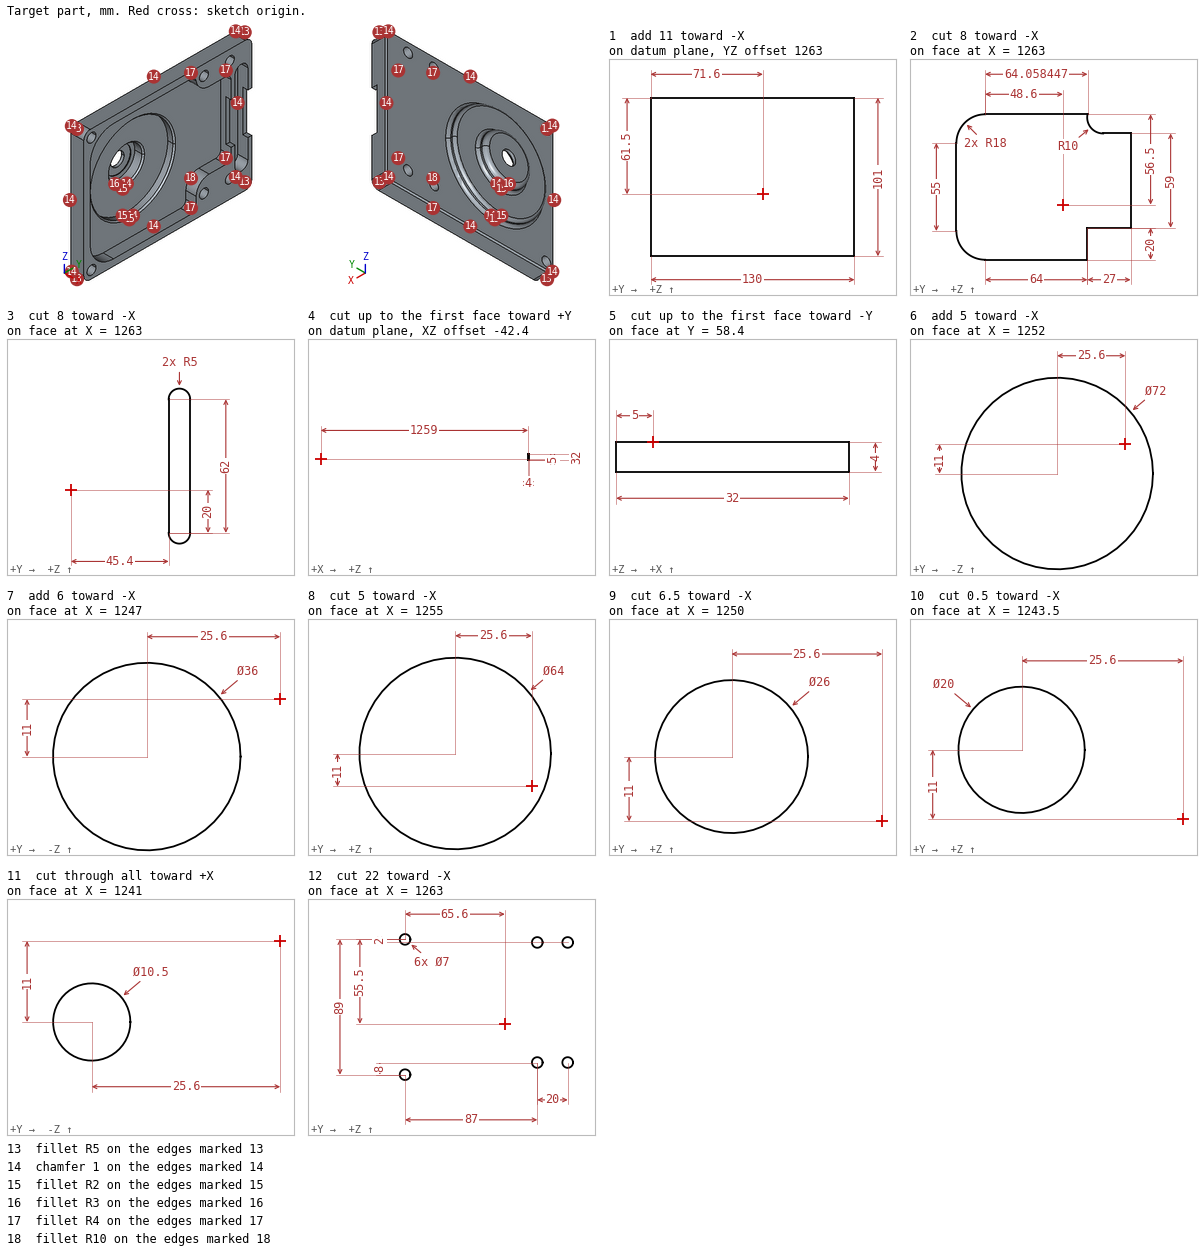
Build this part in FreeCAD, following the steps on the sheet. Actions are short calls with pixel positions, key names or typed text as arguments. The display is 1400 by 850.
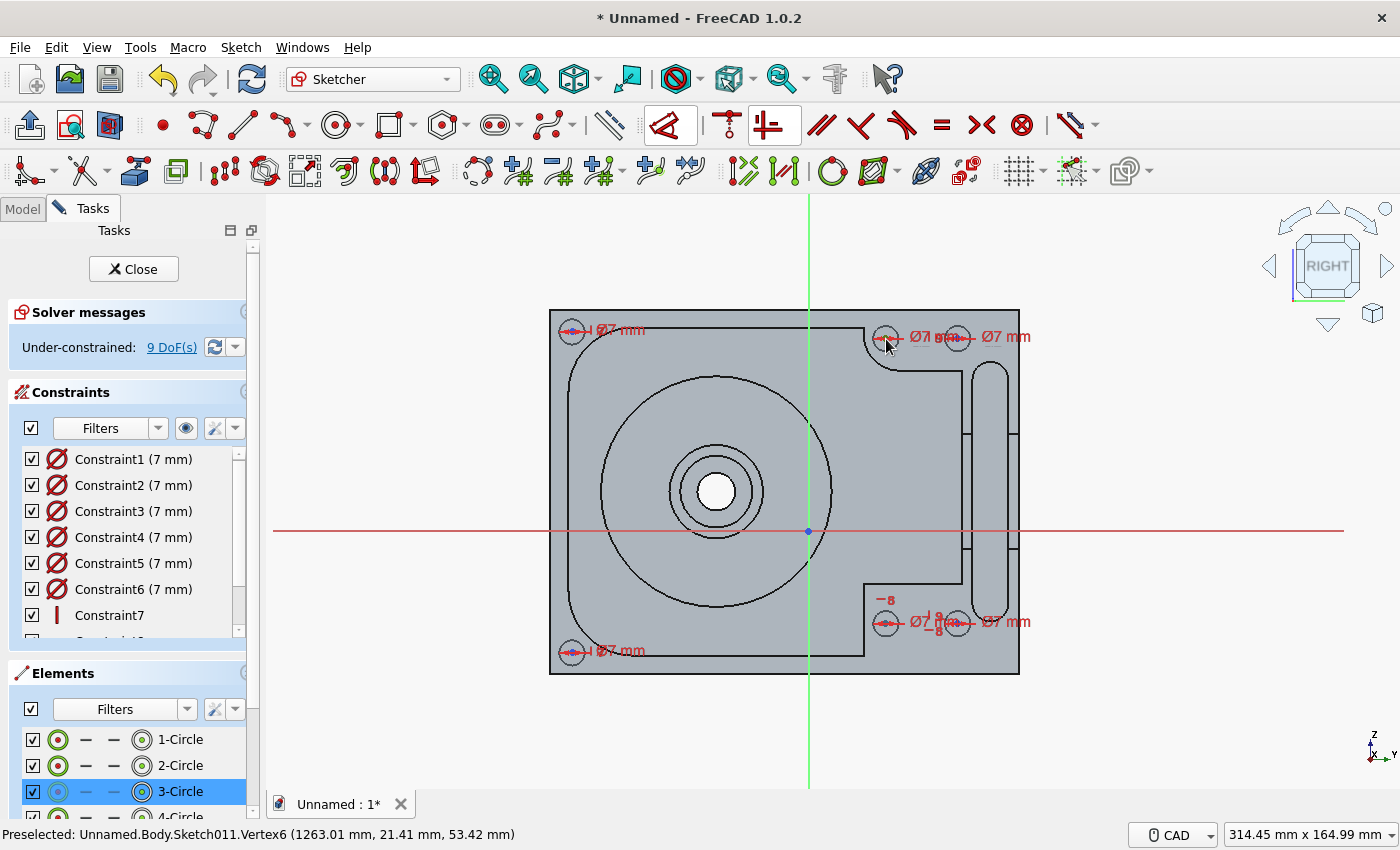
key(v)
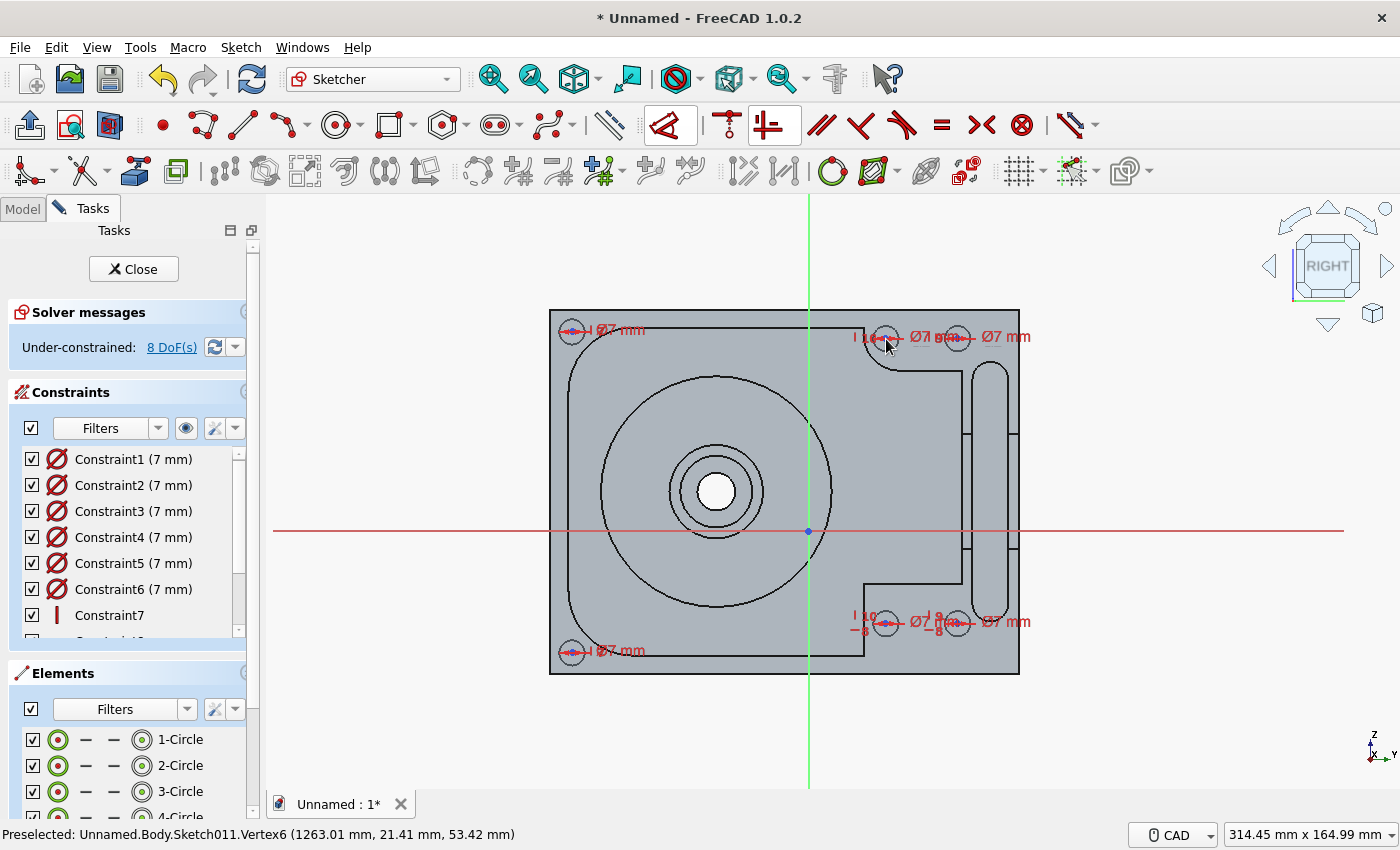
click(958, 339)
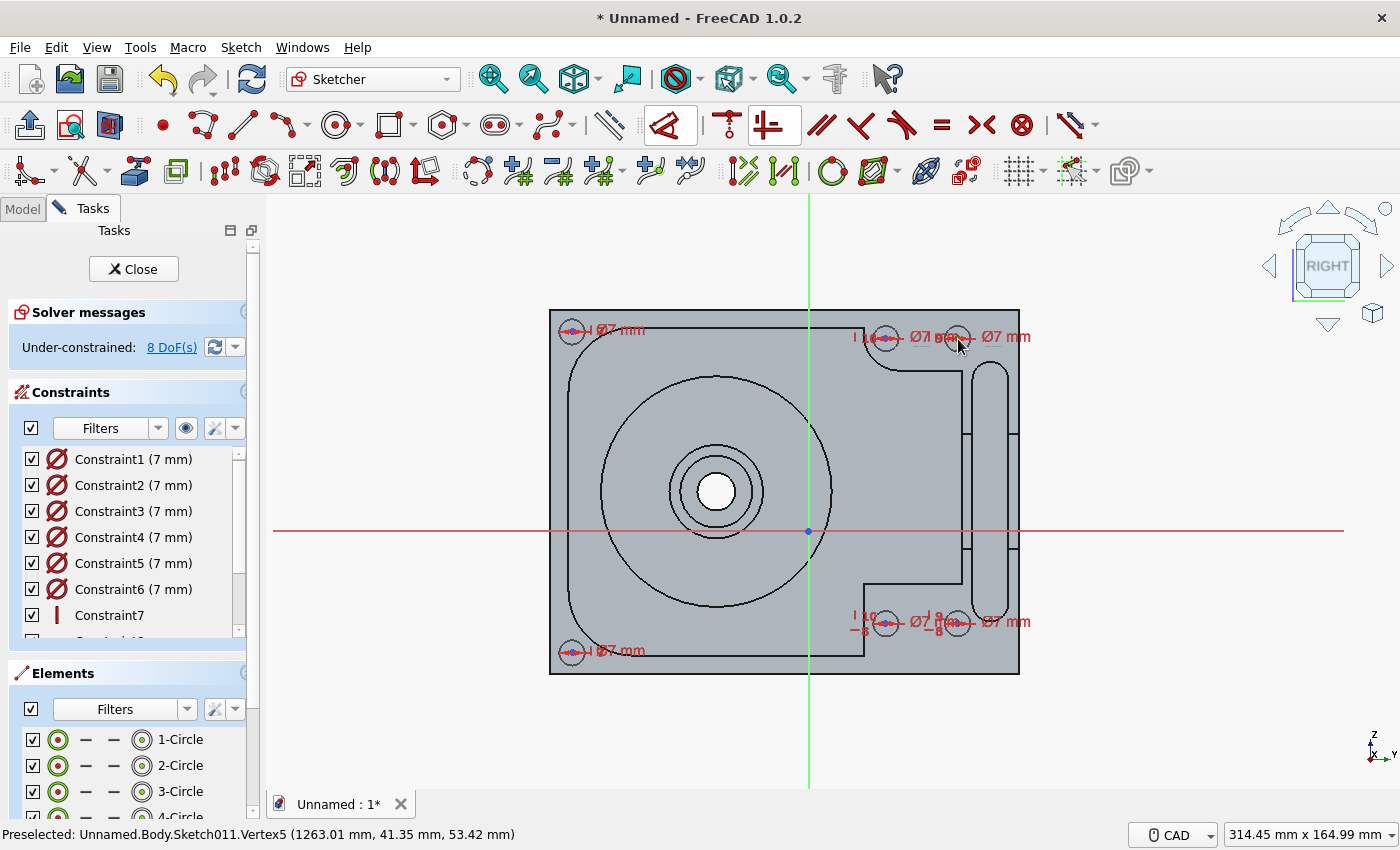
click(886, 339)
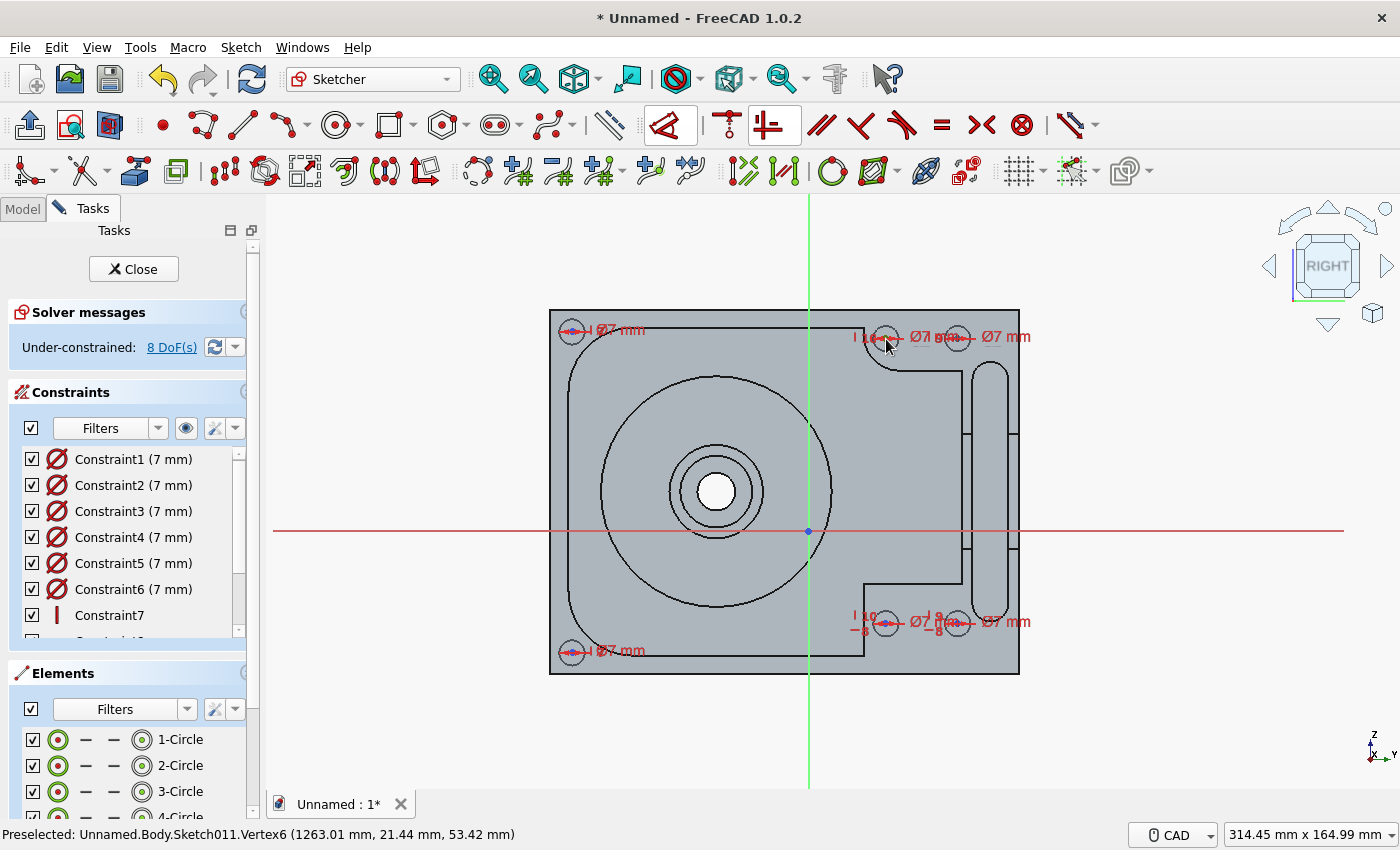
key(h)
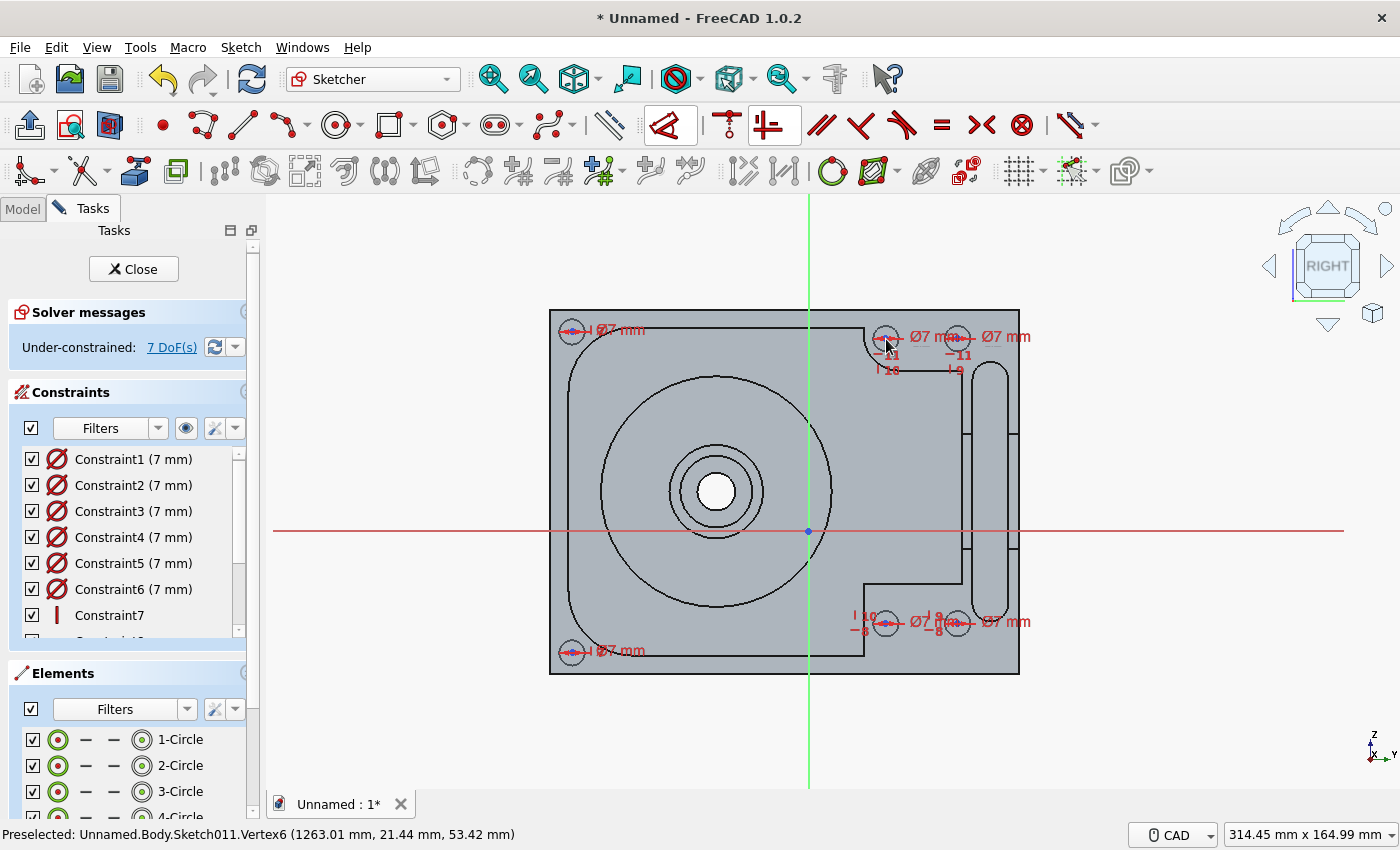
scroll(572, 653, up, 2)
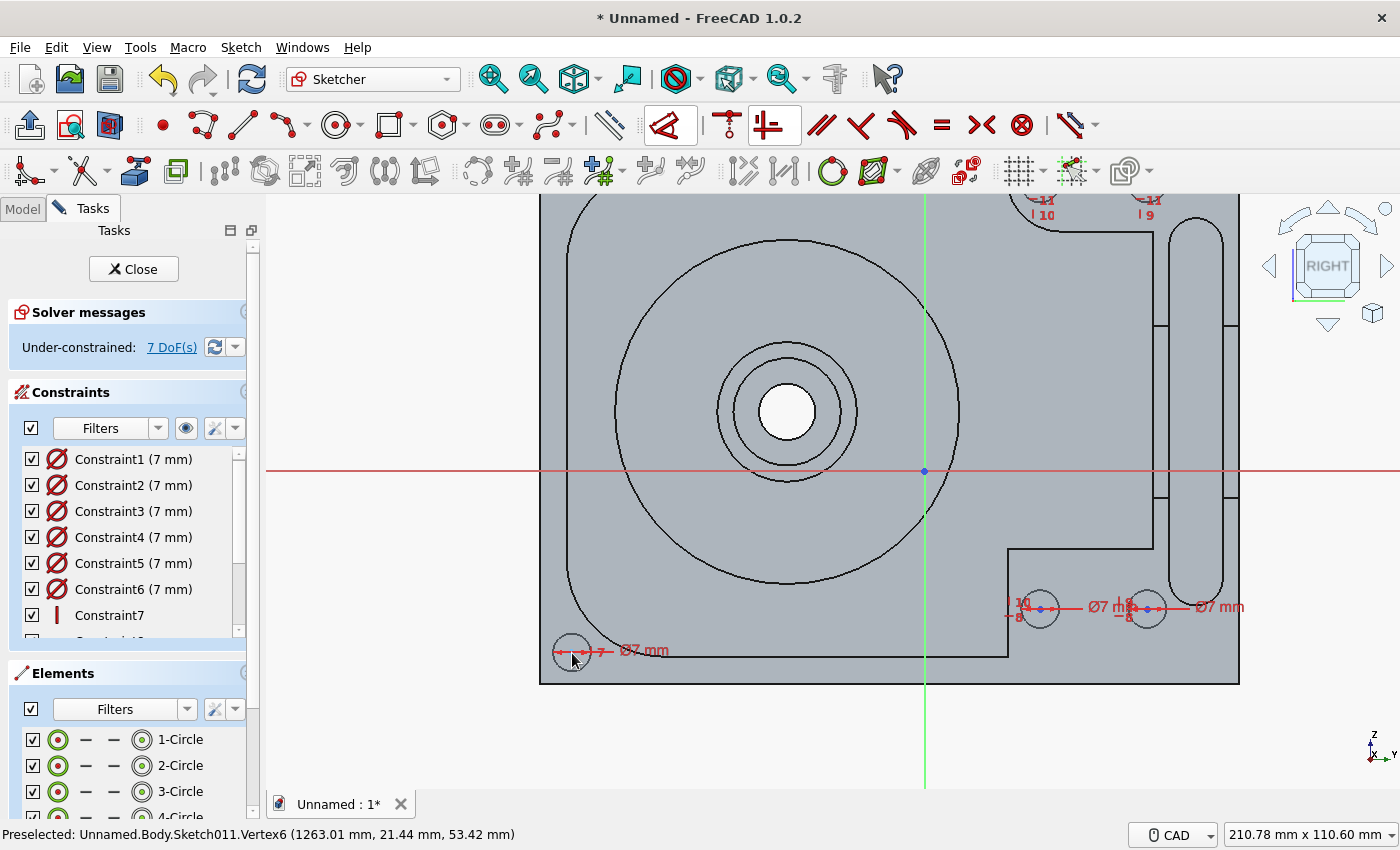
click(572, 652)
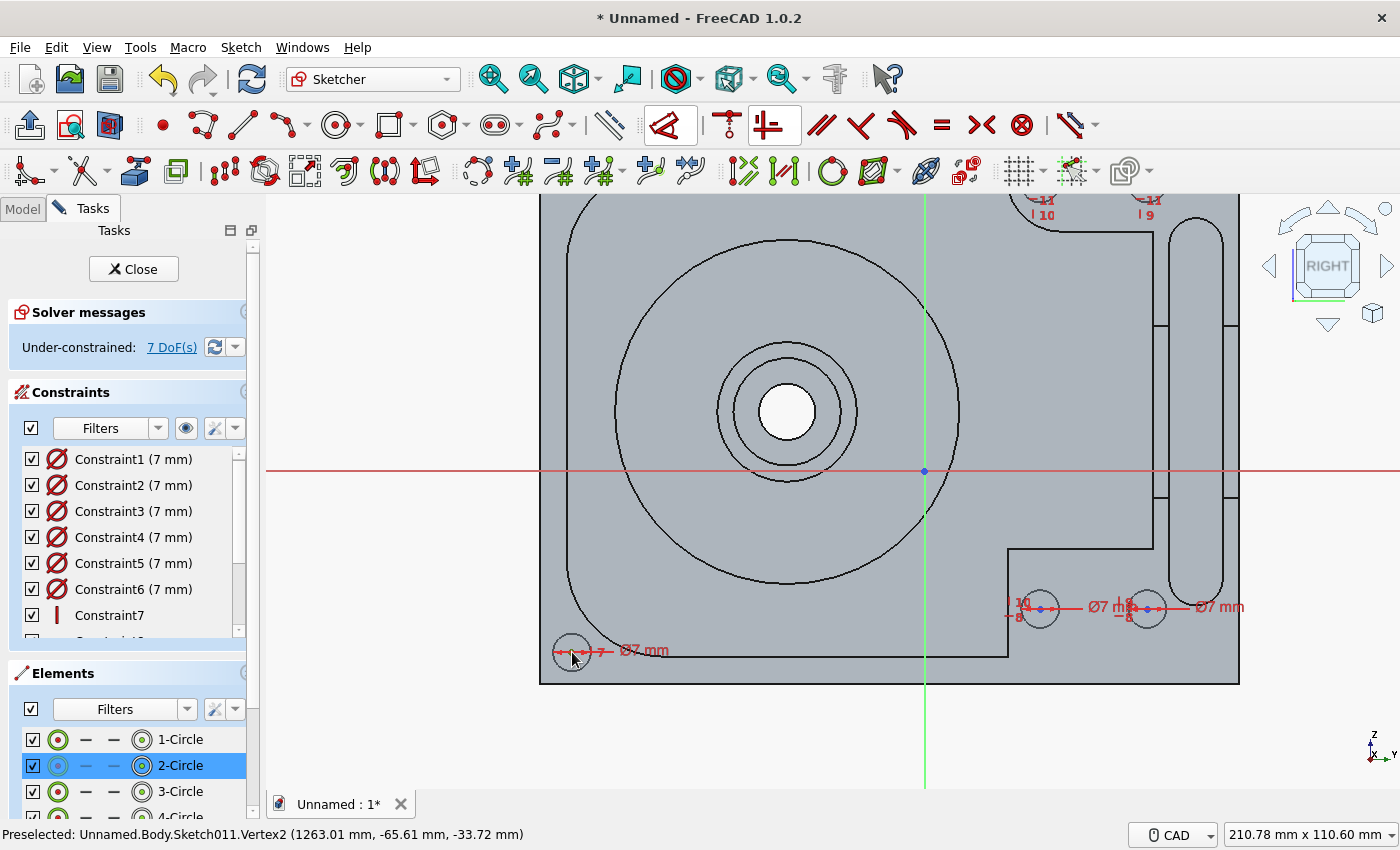
click(1040, 609)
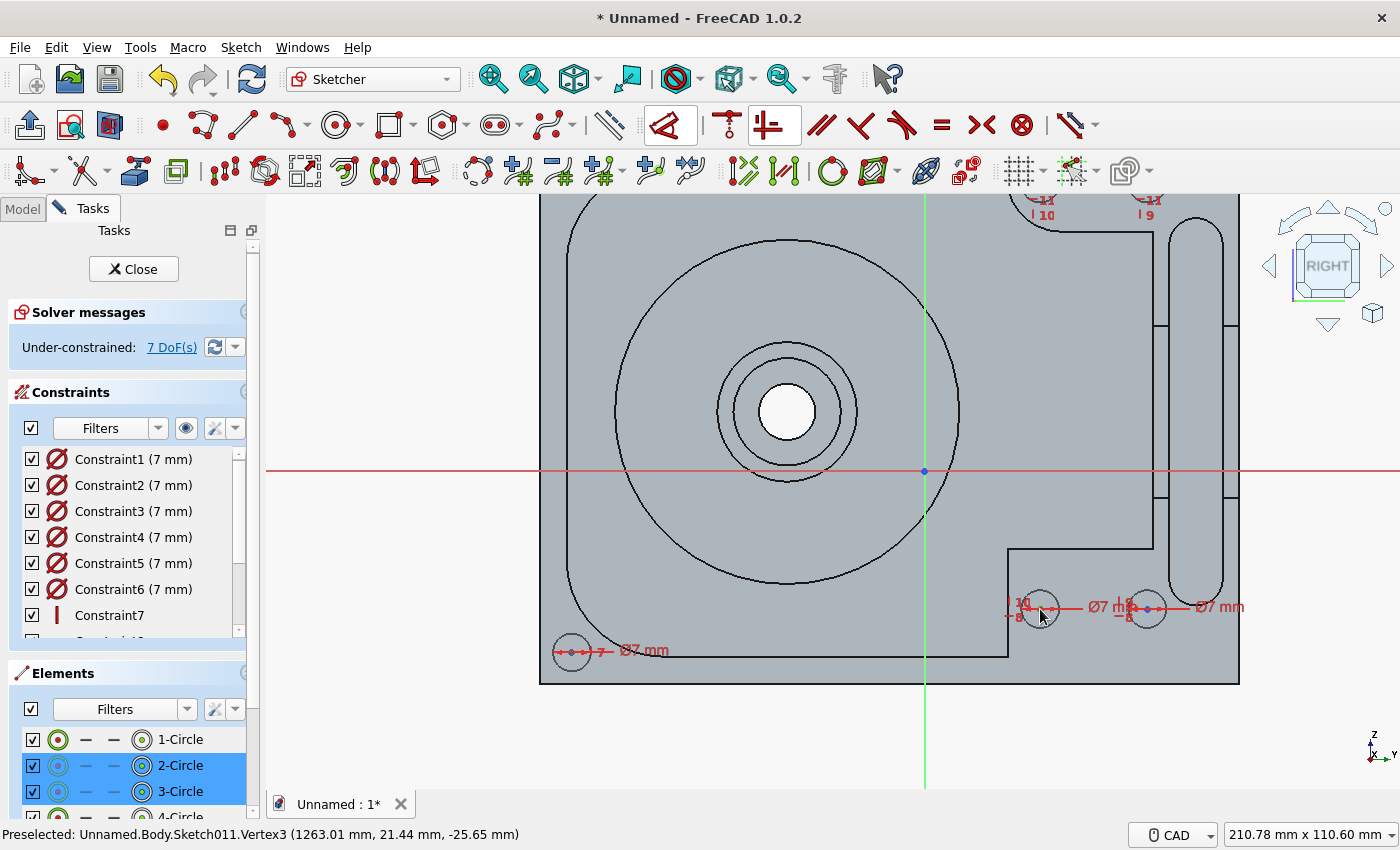
key(i)